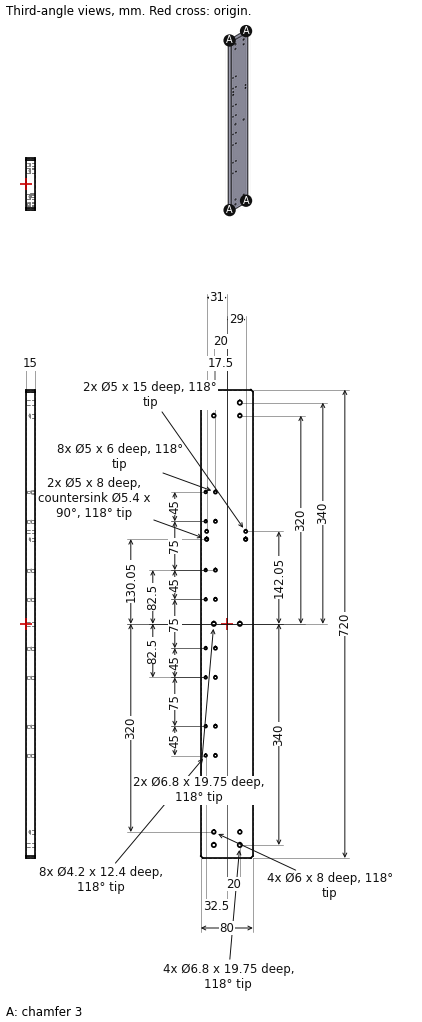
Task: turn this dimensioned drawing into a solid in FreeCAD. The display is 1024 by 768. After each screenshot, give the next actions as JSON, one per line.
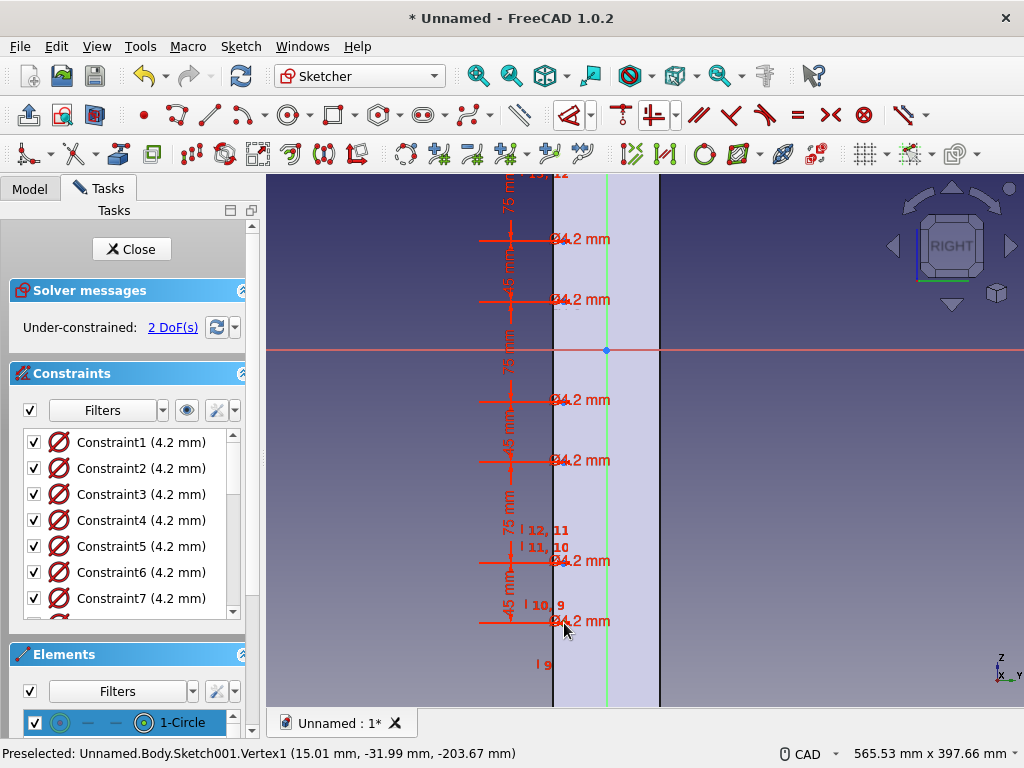
{"action": "left_click", "coordinate": [590, 116]}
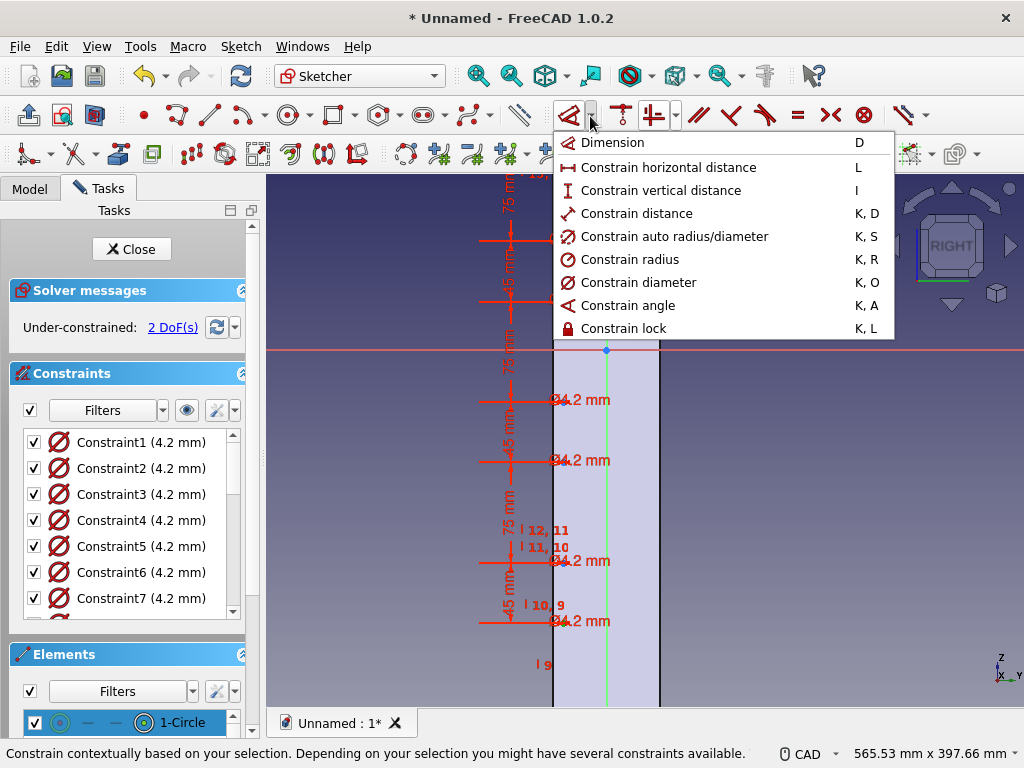
{"action": "left_click", "coordinate": [724, 168]}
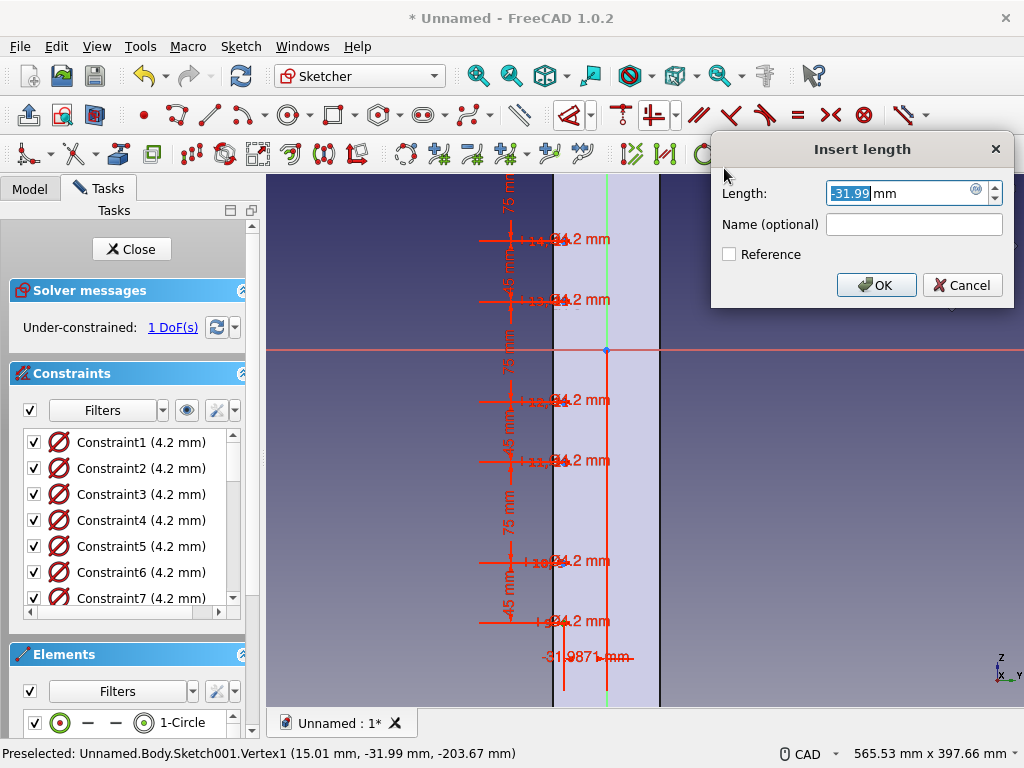
{"action": "type", "text": "-32.5"}
{"action": "key", "text": "Return"}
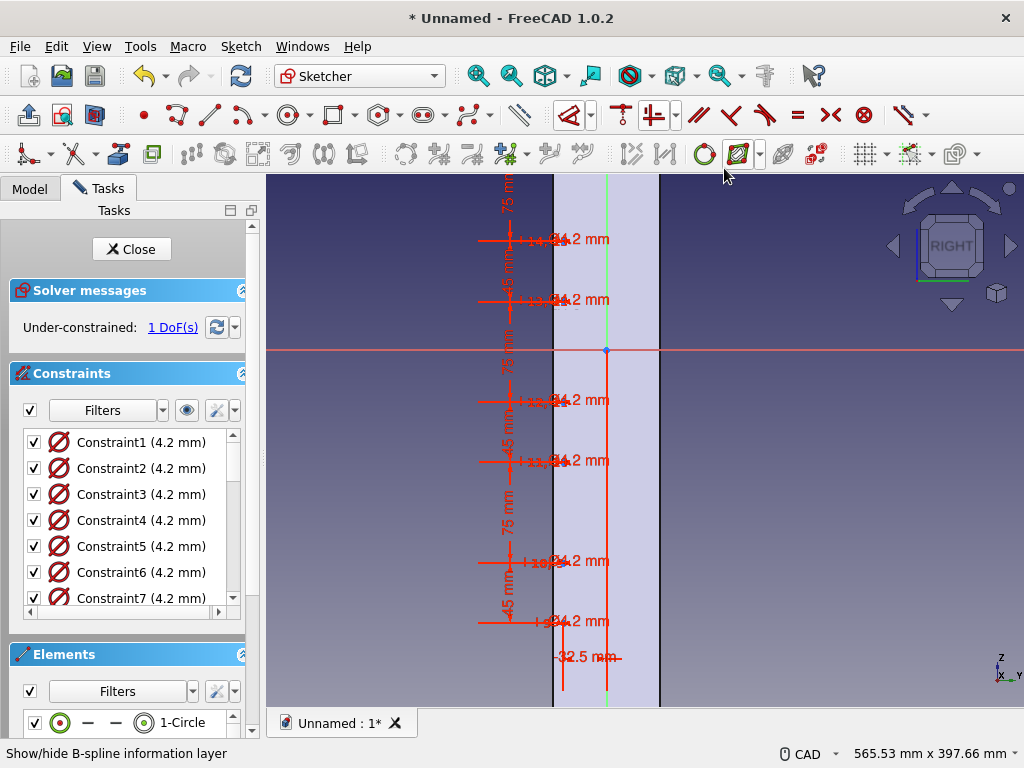
{"action": "left_click", "coordinate": [563, 462]}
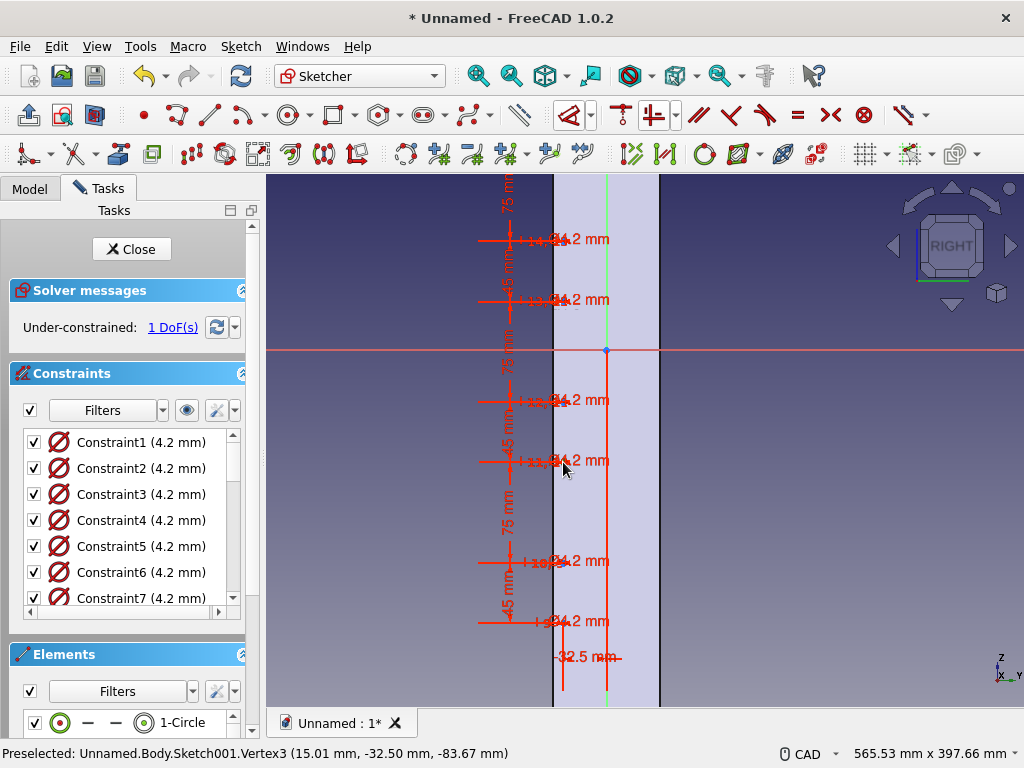
{"action": "left_click", "coordinate": [590, 116]}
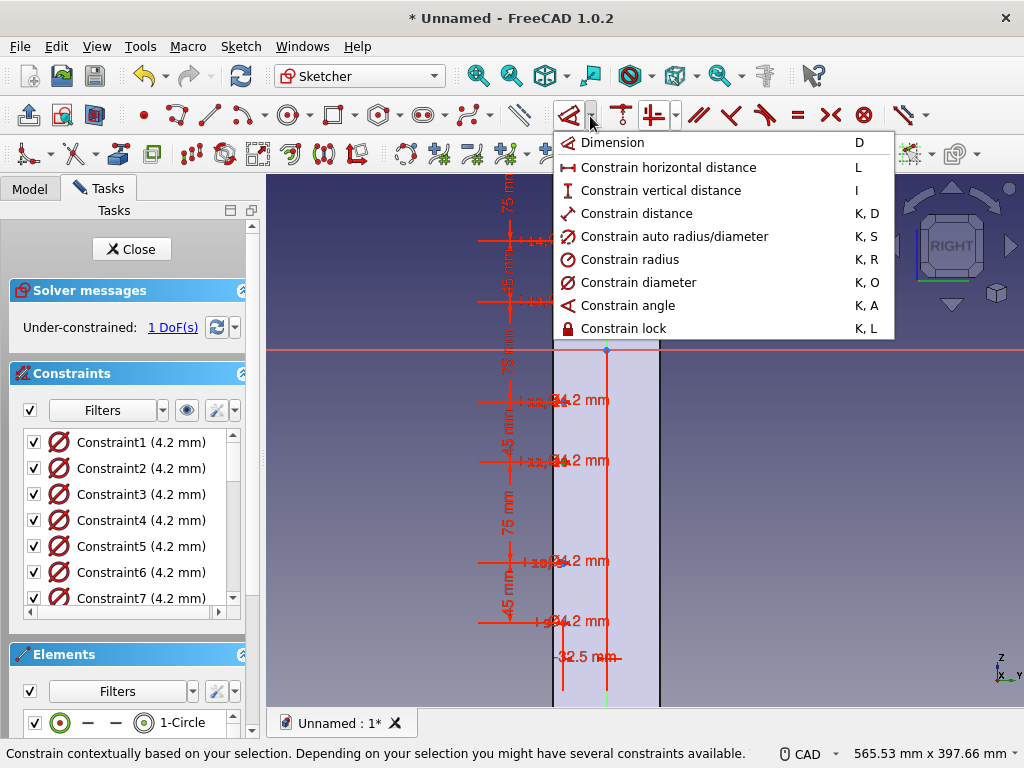
{"action": "left_click", "coordinate": [724, 190]}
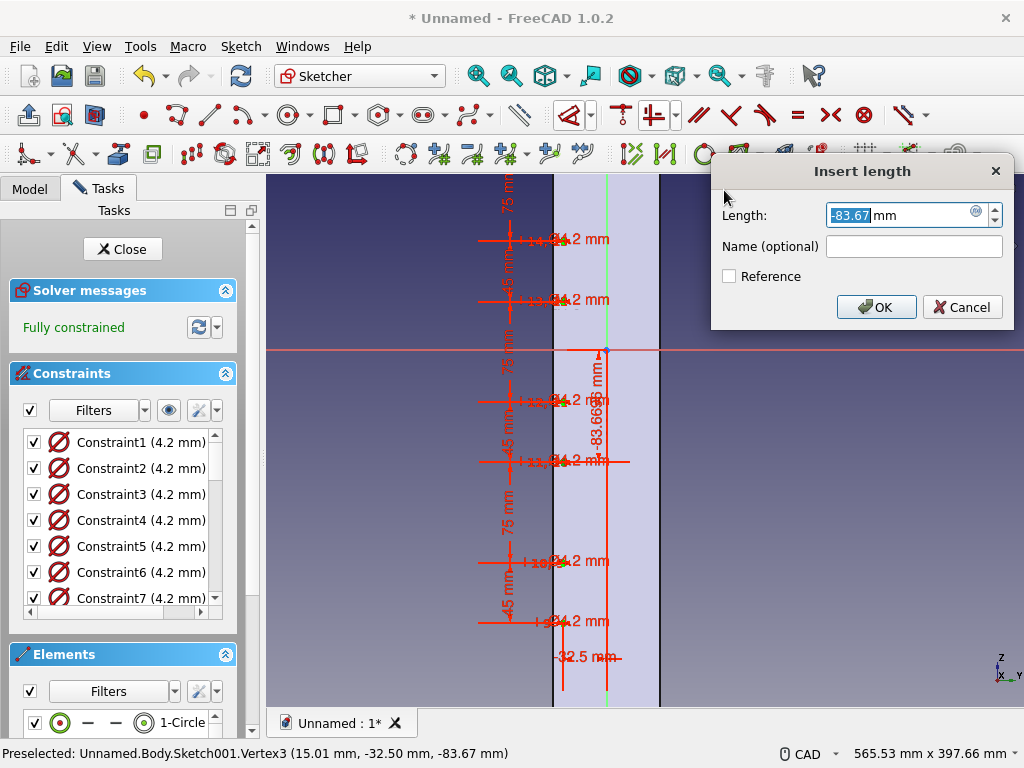
{"action": "type", "text": "-82.5"}
{"action": "key", "text": "Return"}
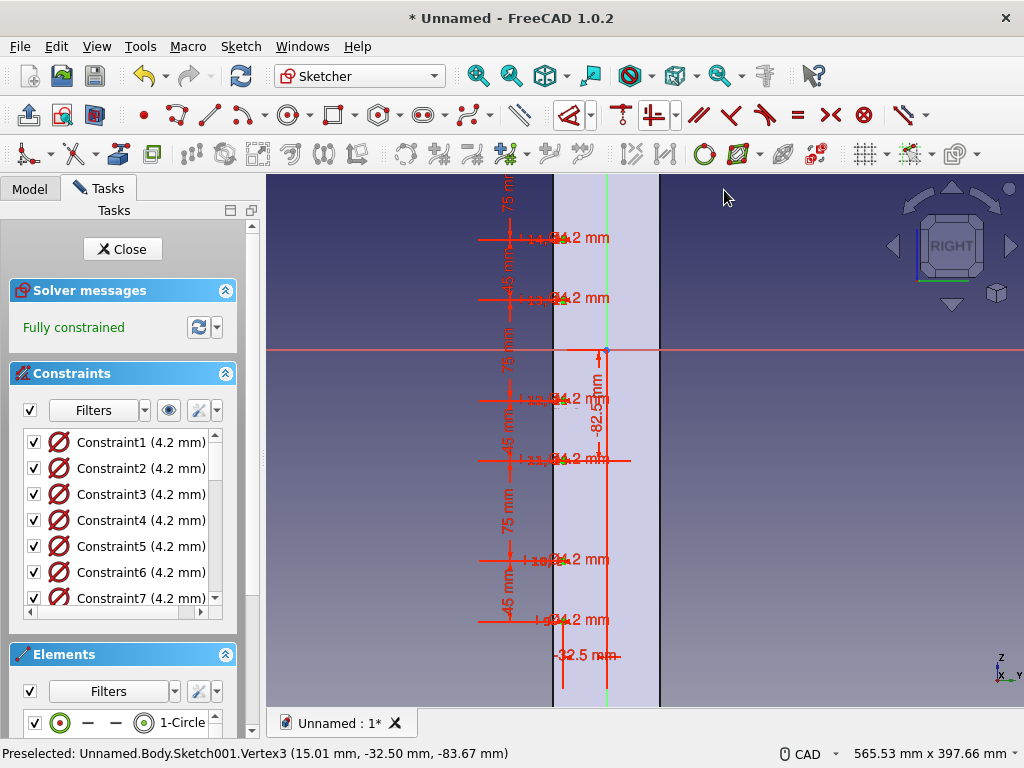
{"action": "left_click", "coordinate": [123, 249]}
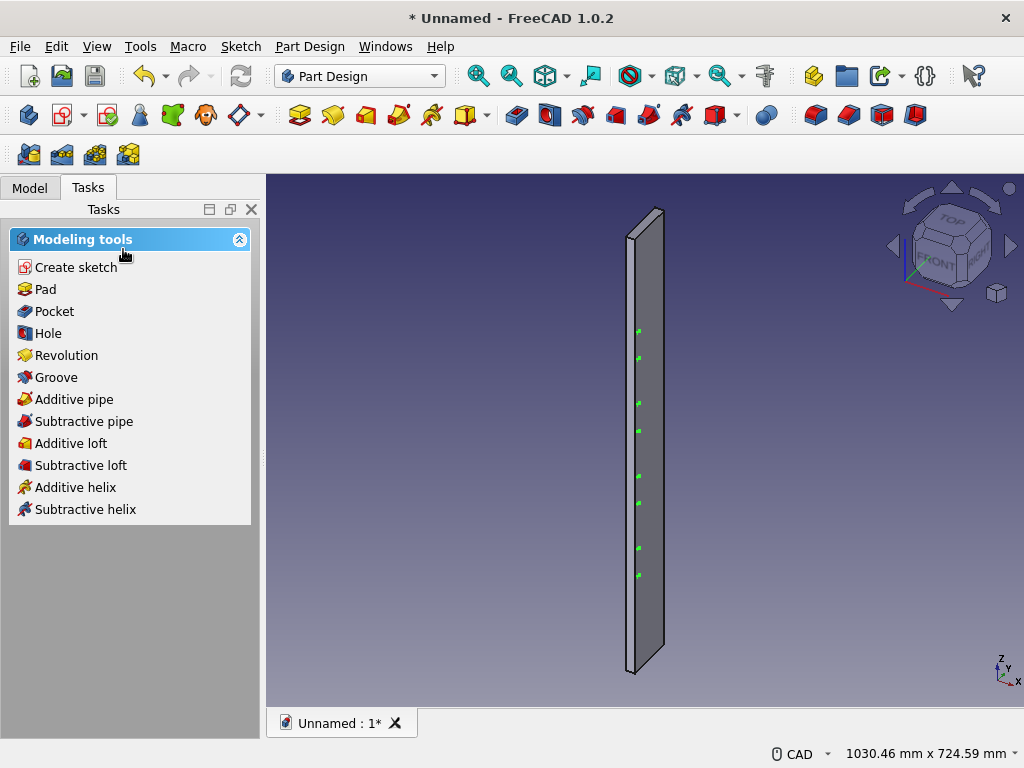
{"action": "left_click", "coordinate": [550, 116]}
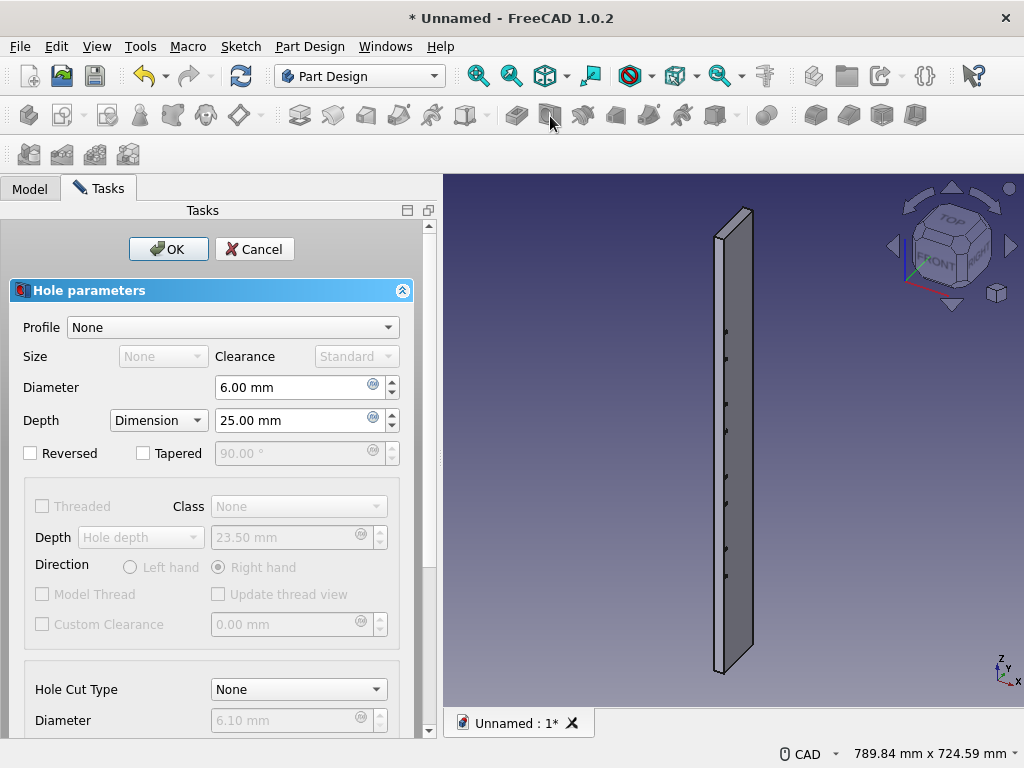
{"action": "triple_click", "coordinate": [300, 388]}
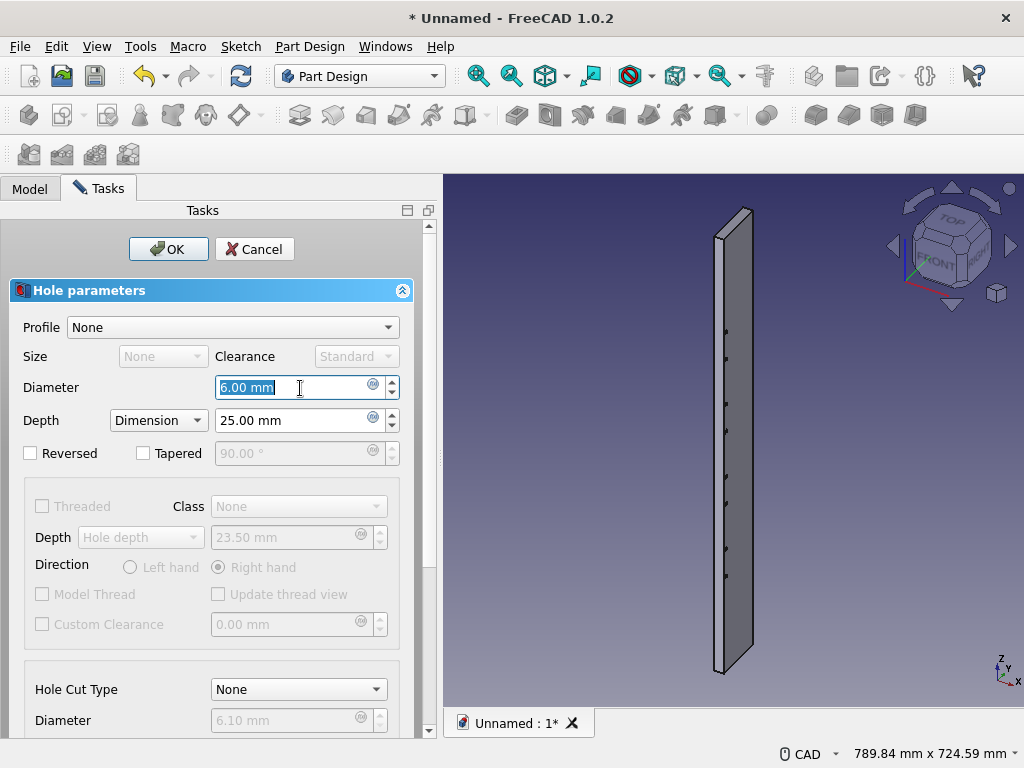
{"action": "type", "text": "4.2"}
{"action": "key", "text": "Tab"}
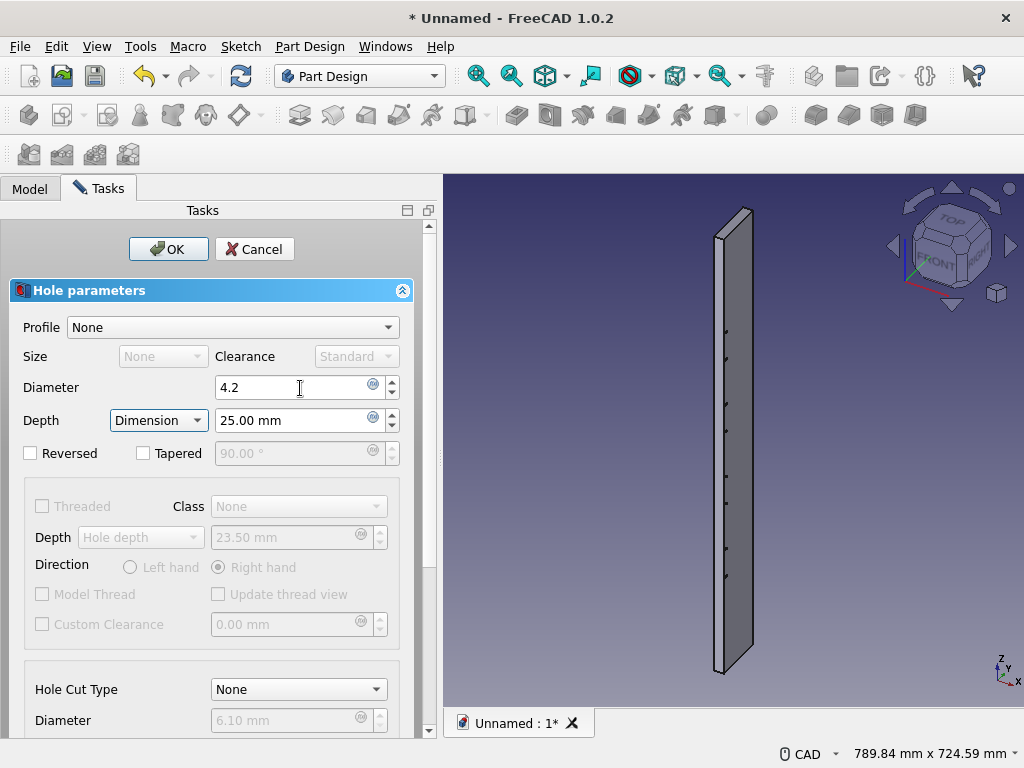
{"action": "triple_click", "coordinate": [300, 420]}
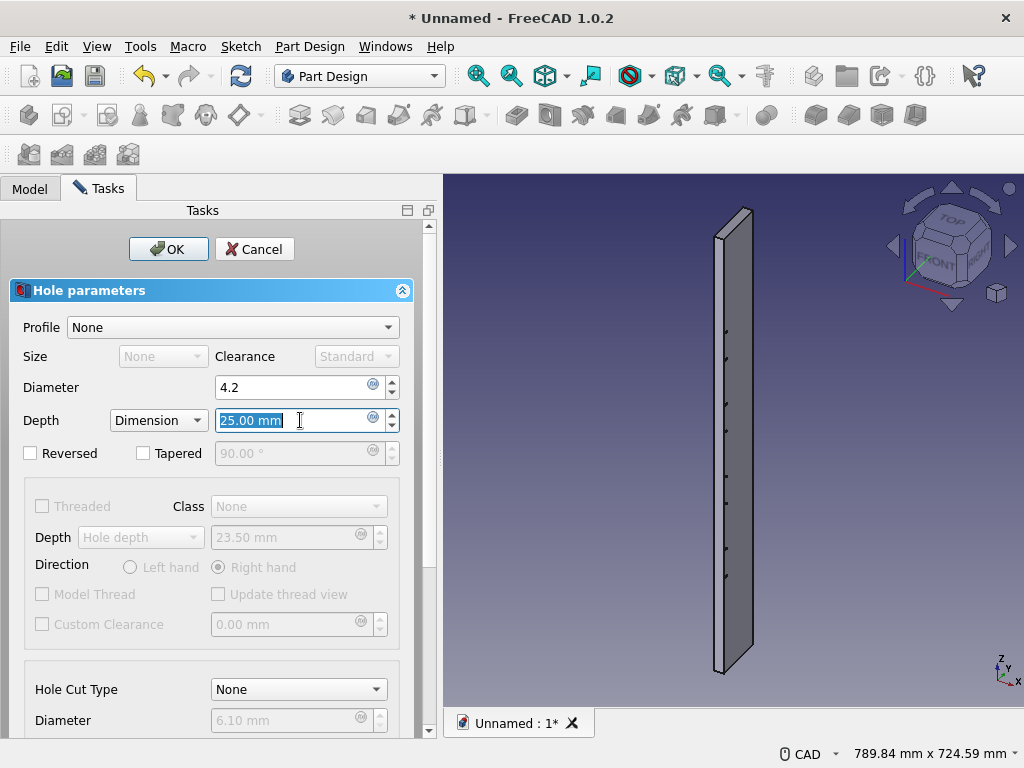
{"action": "type", "text": "12.4"}
{"action": "key", "text": "Tab"}